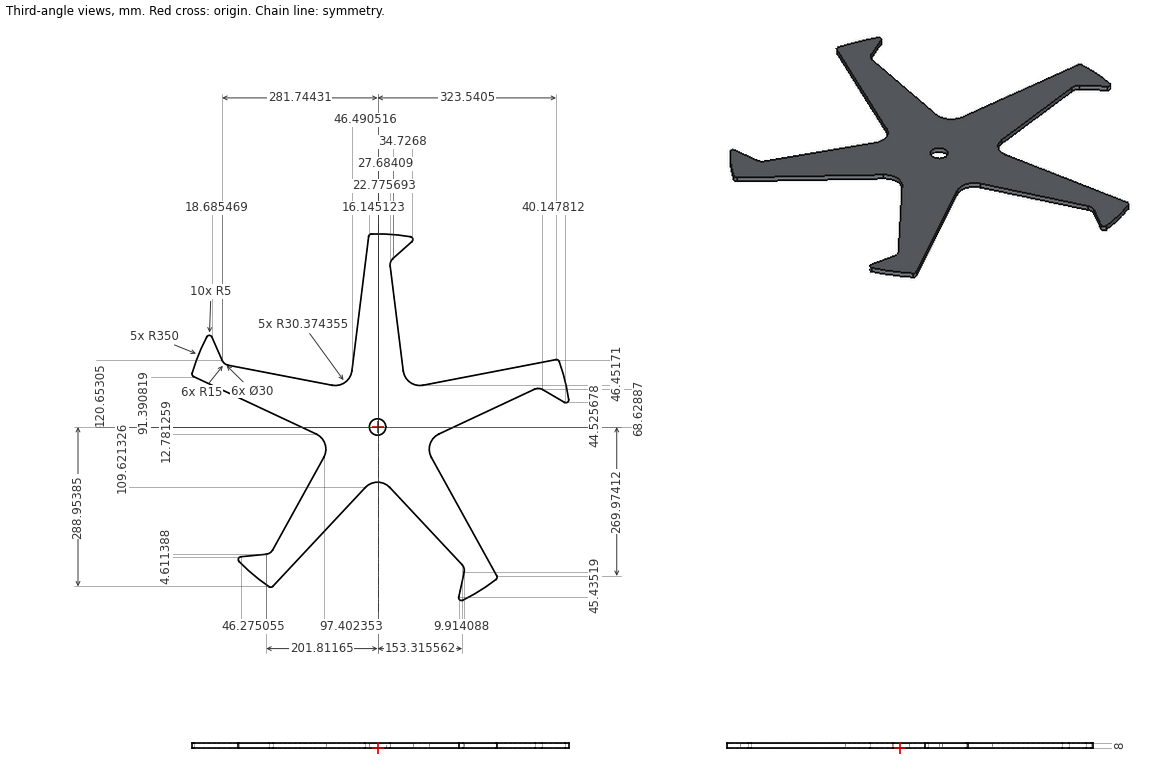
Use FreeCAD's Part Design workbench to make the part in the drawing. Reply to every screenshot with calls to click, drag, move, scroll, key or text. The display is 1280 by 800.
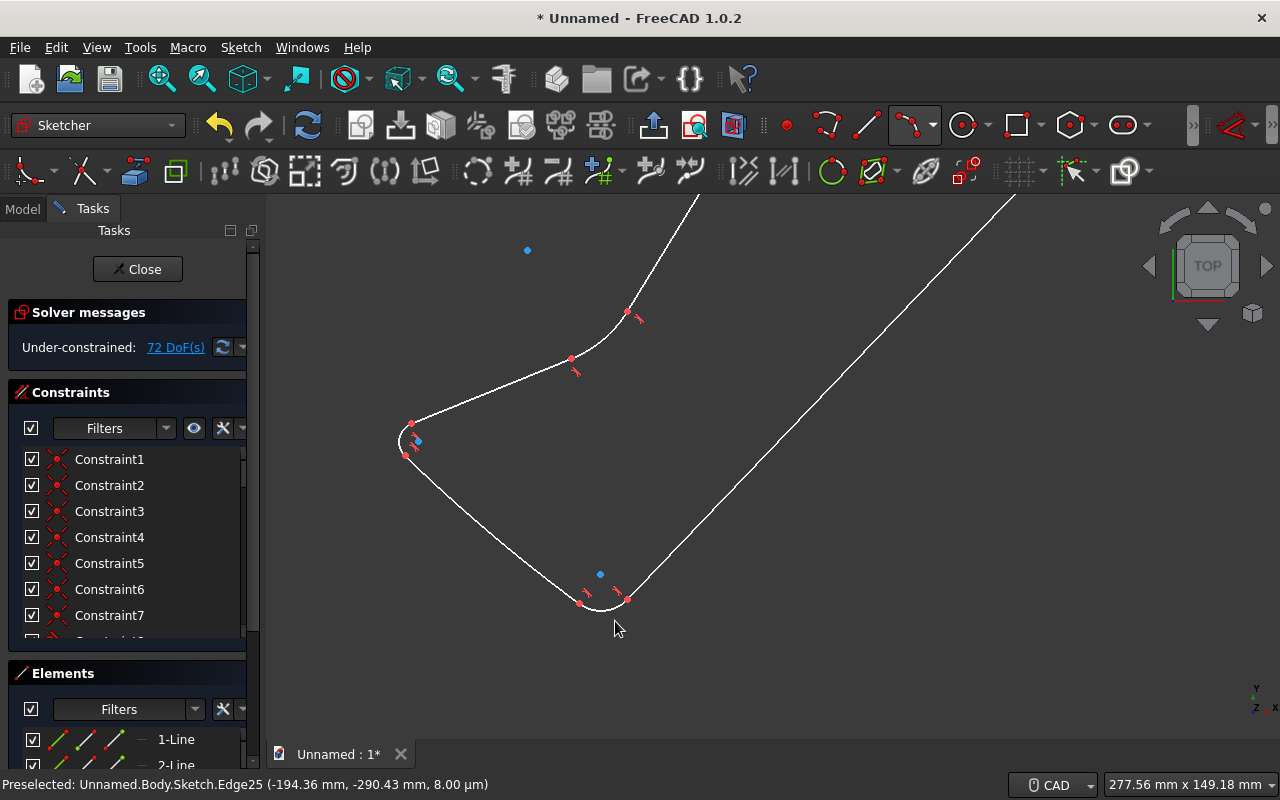
scroll(605, 618, down, 10)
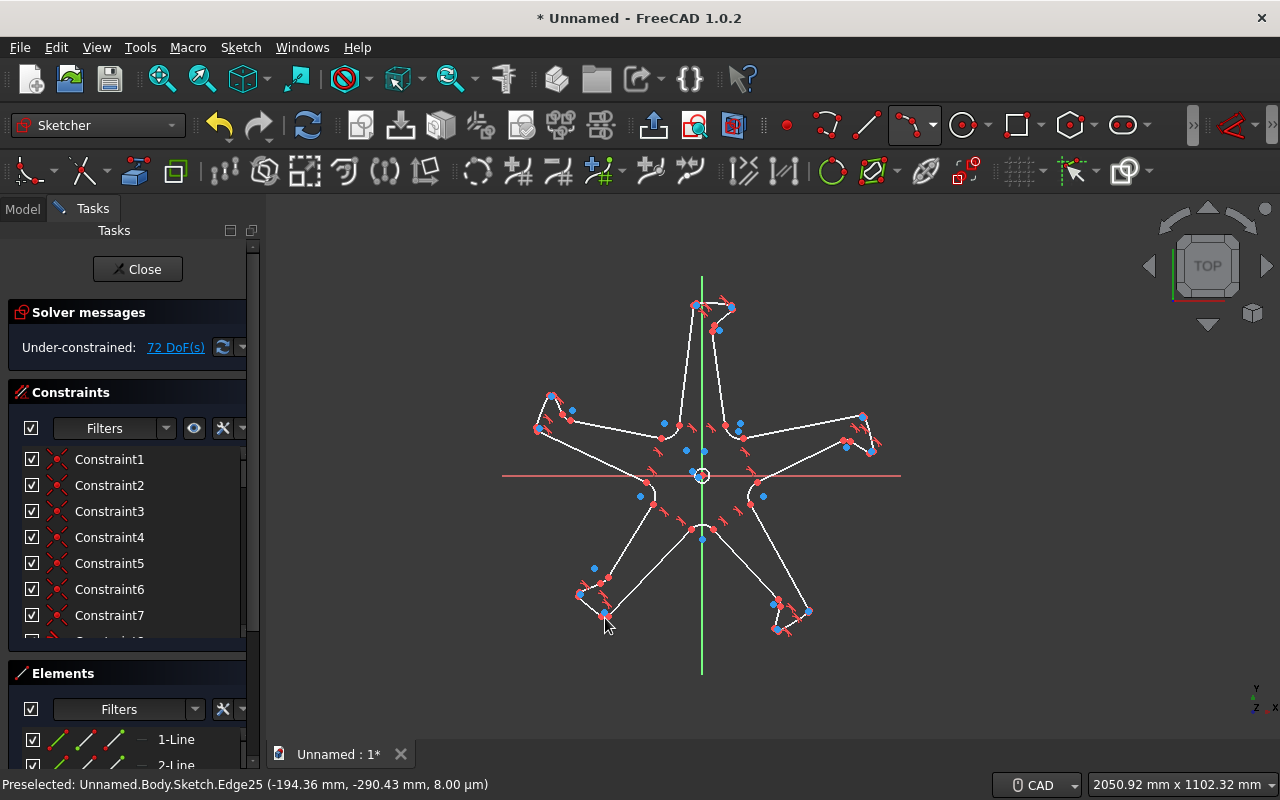
scroll(775, 630, up, 11)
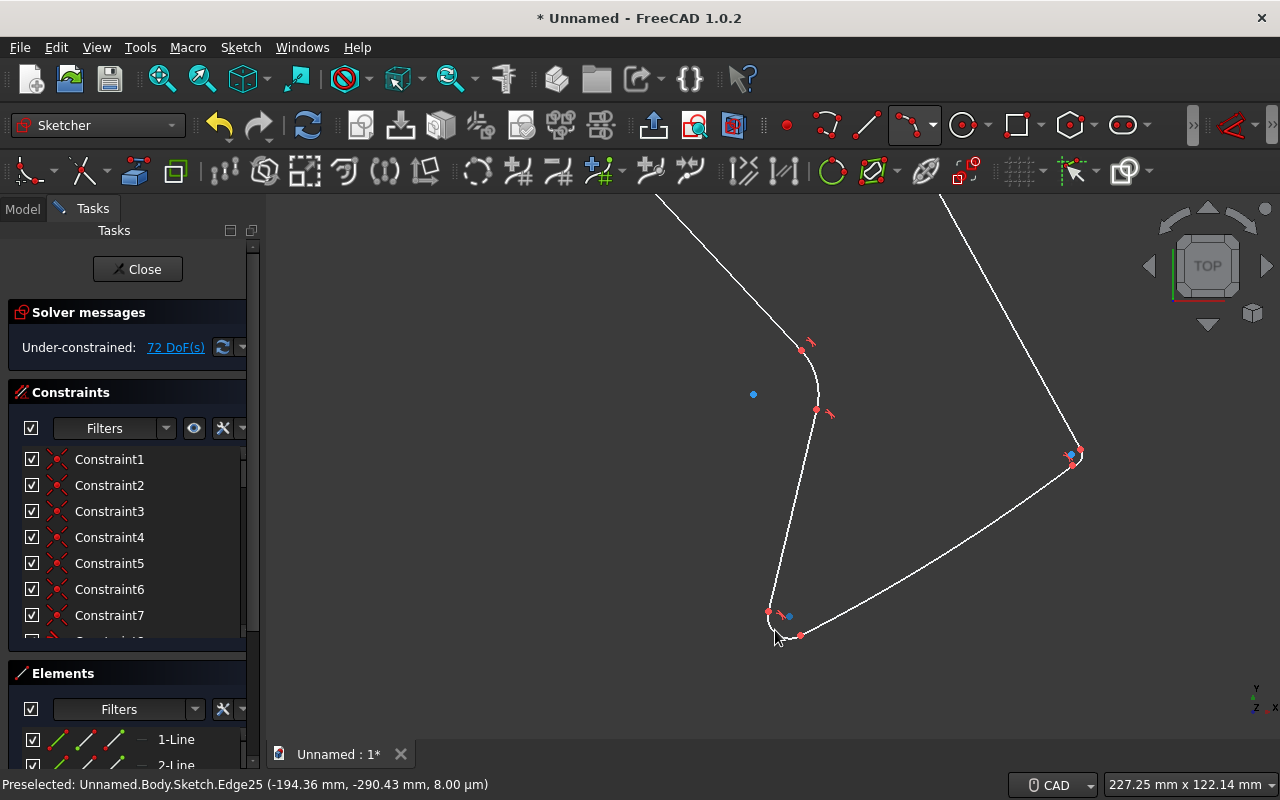
click(770, 627)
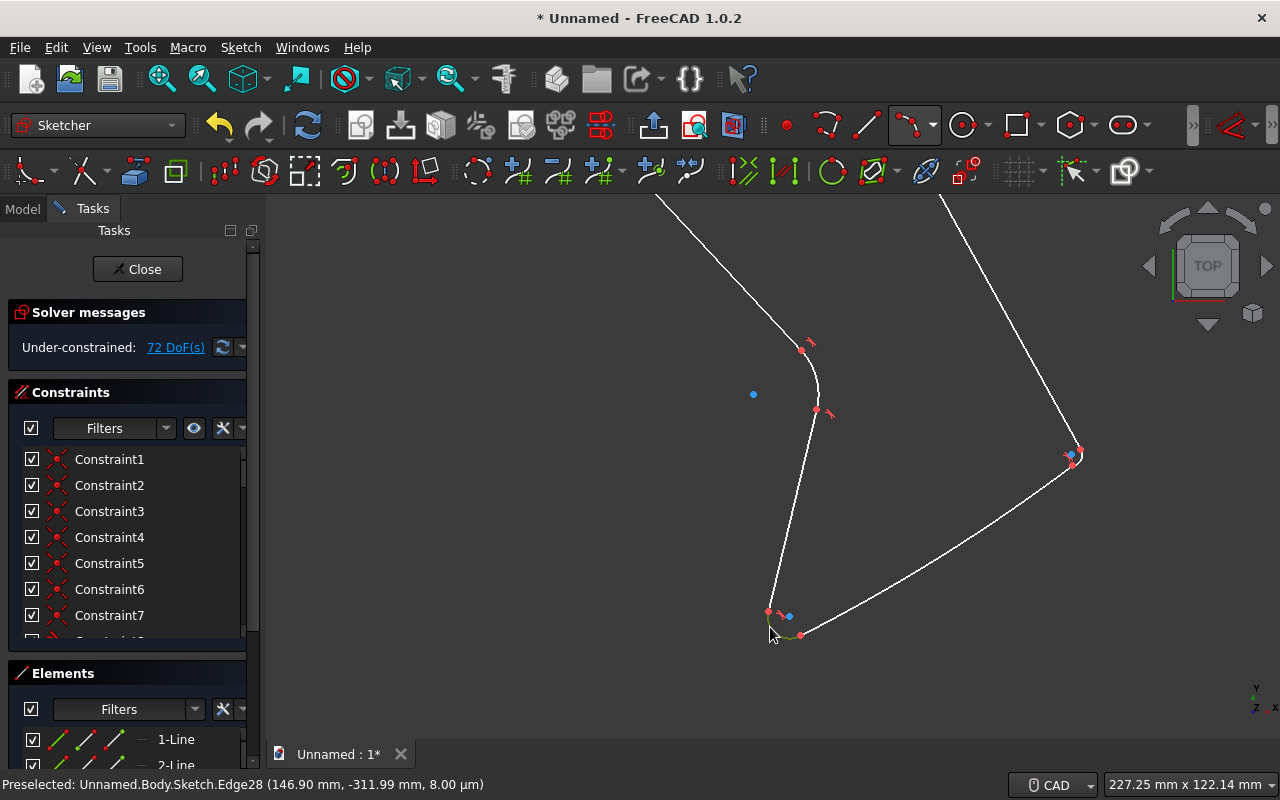
scroll(775, 630, down, 11)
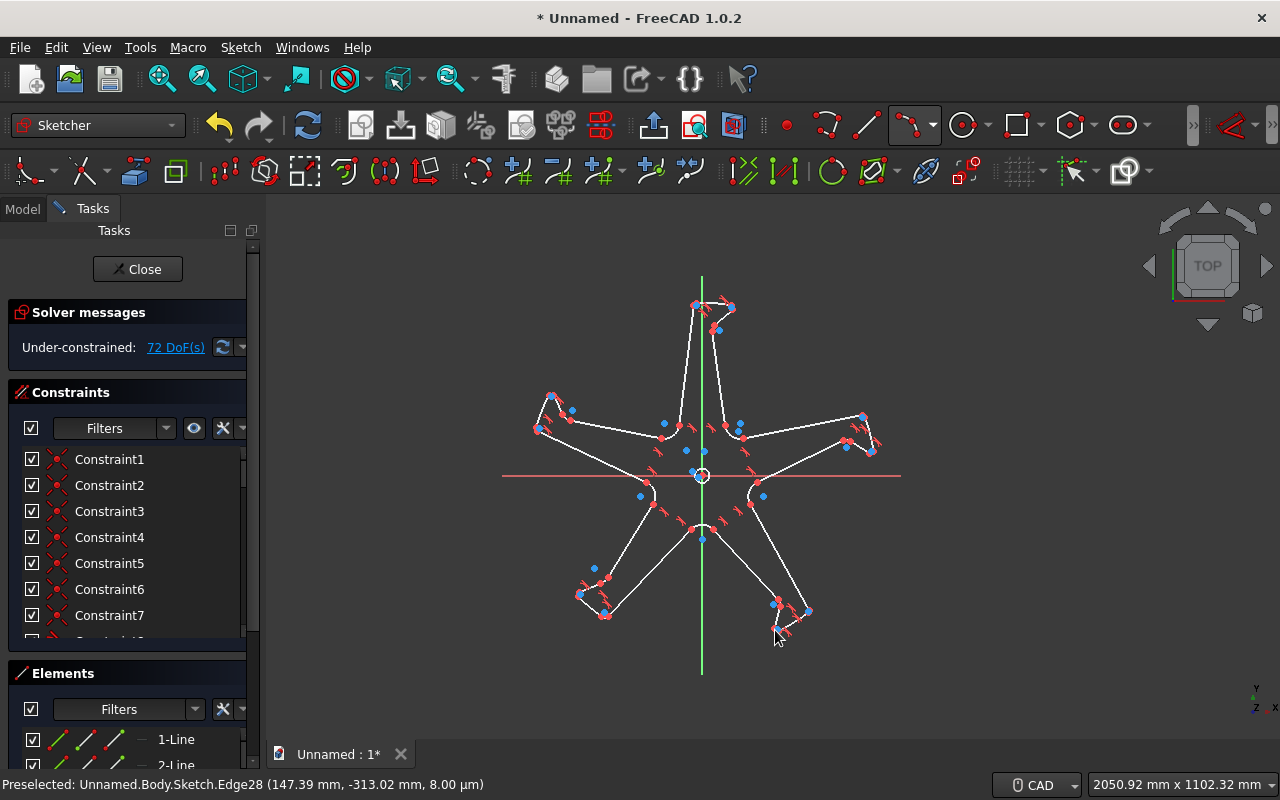
scroll(788, 626, up, 2)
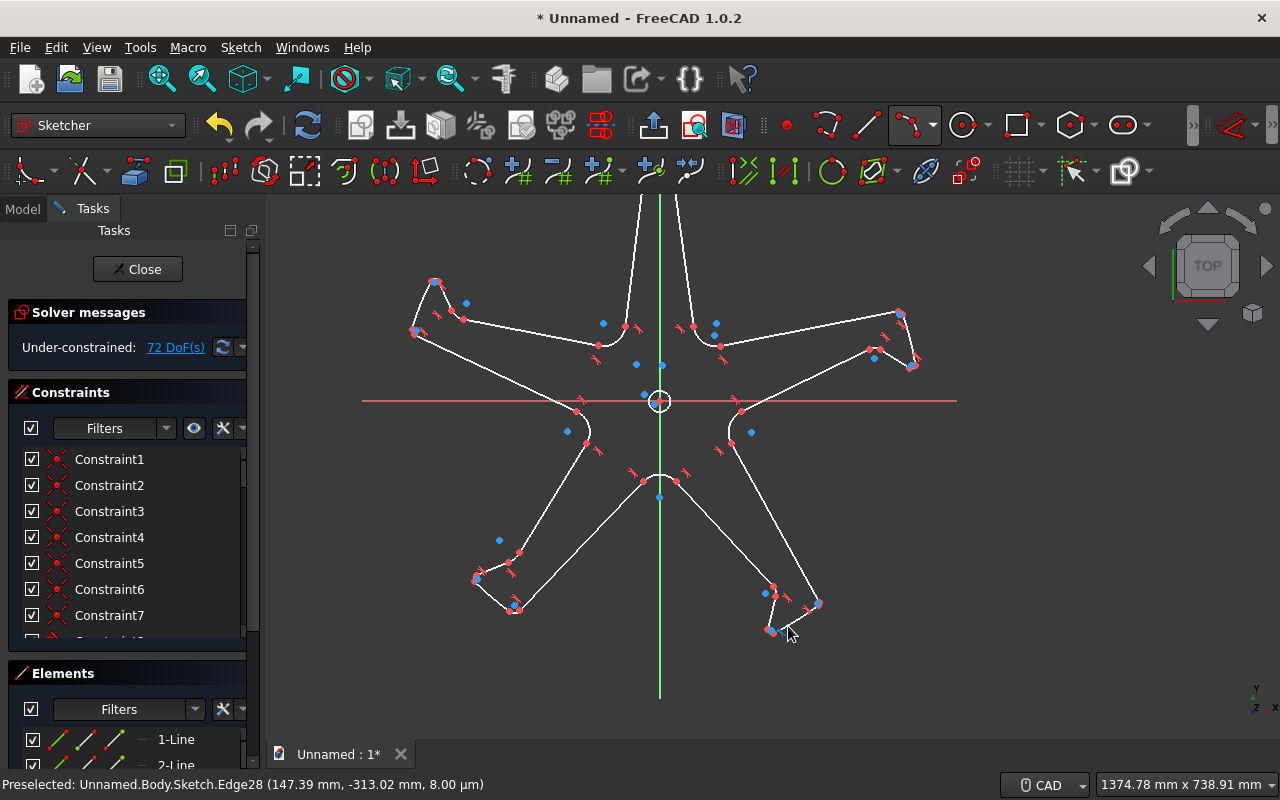
click(805, 615)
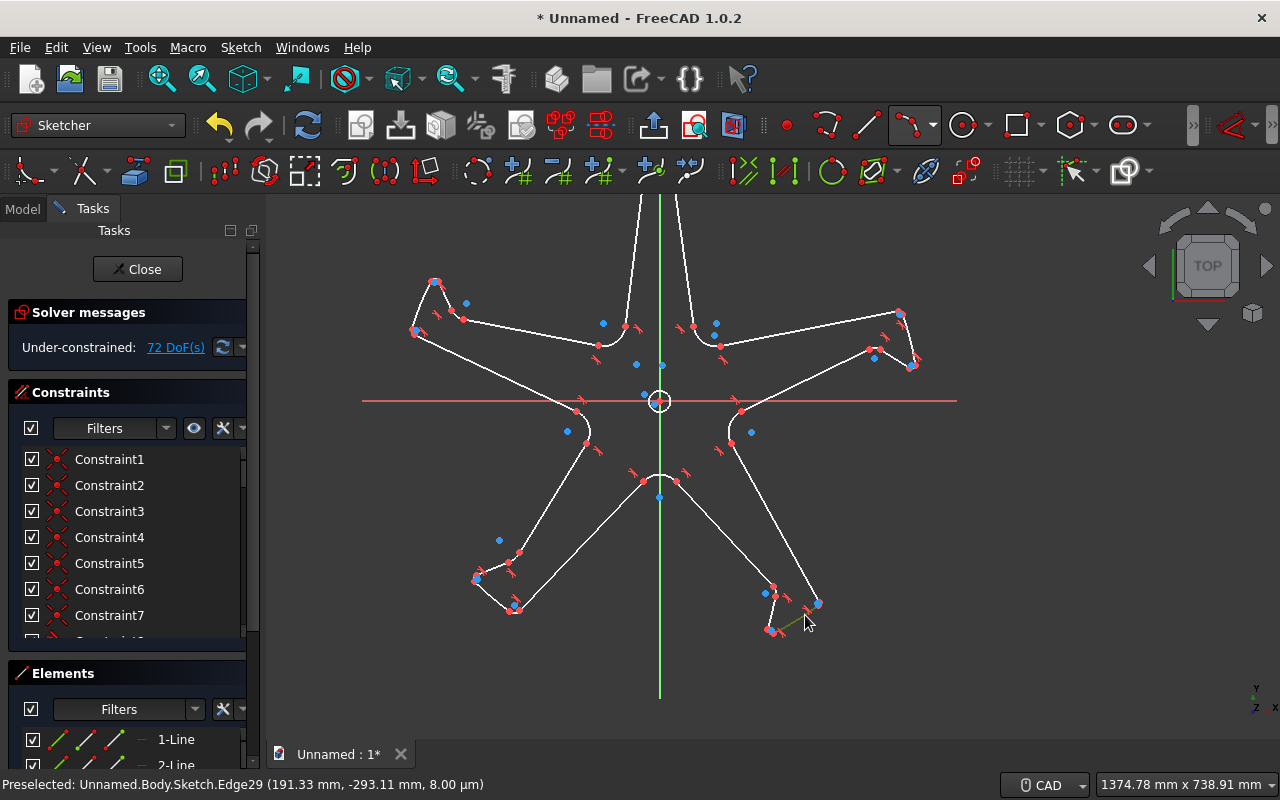
key(t)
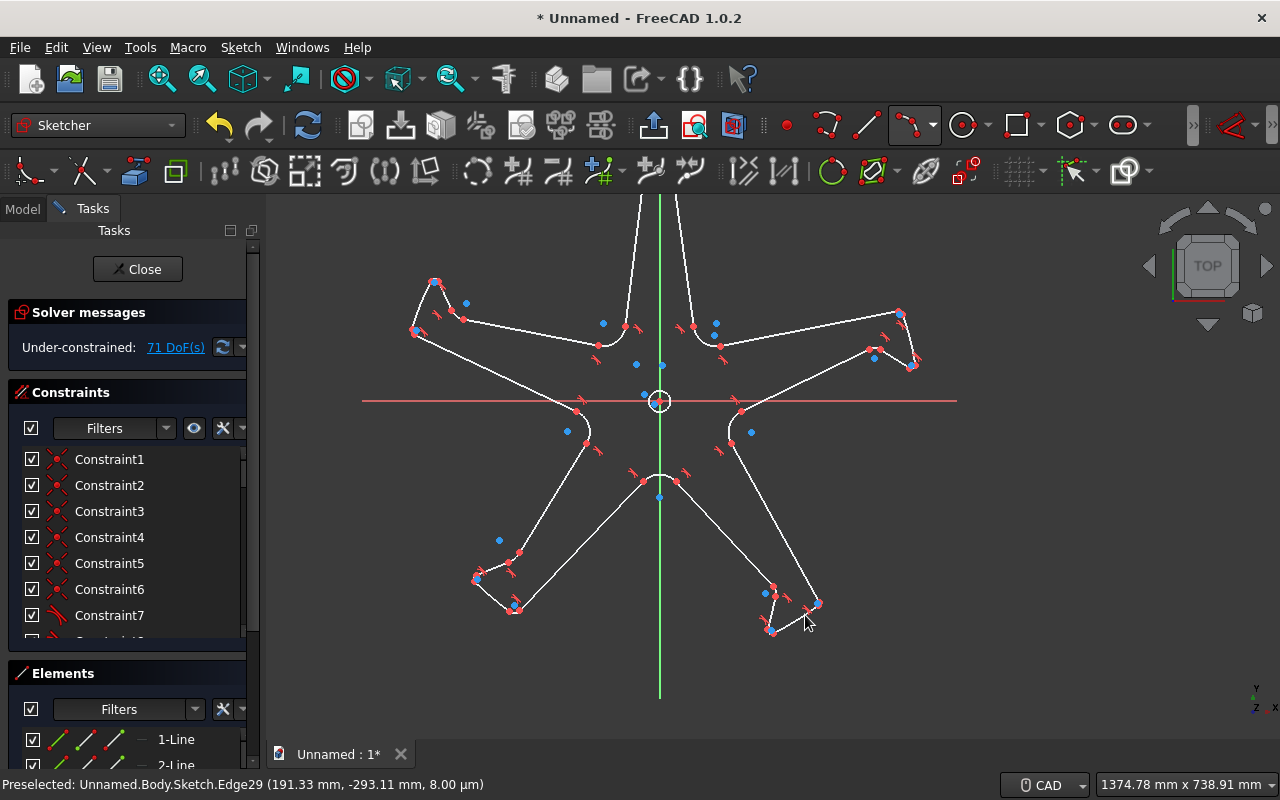
click(787, 626)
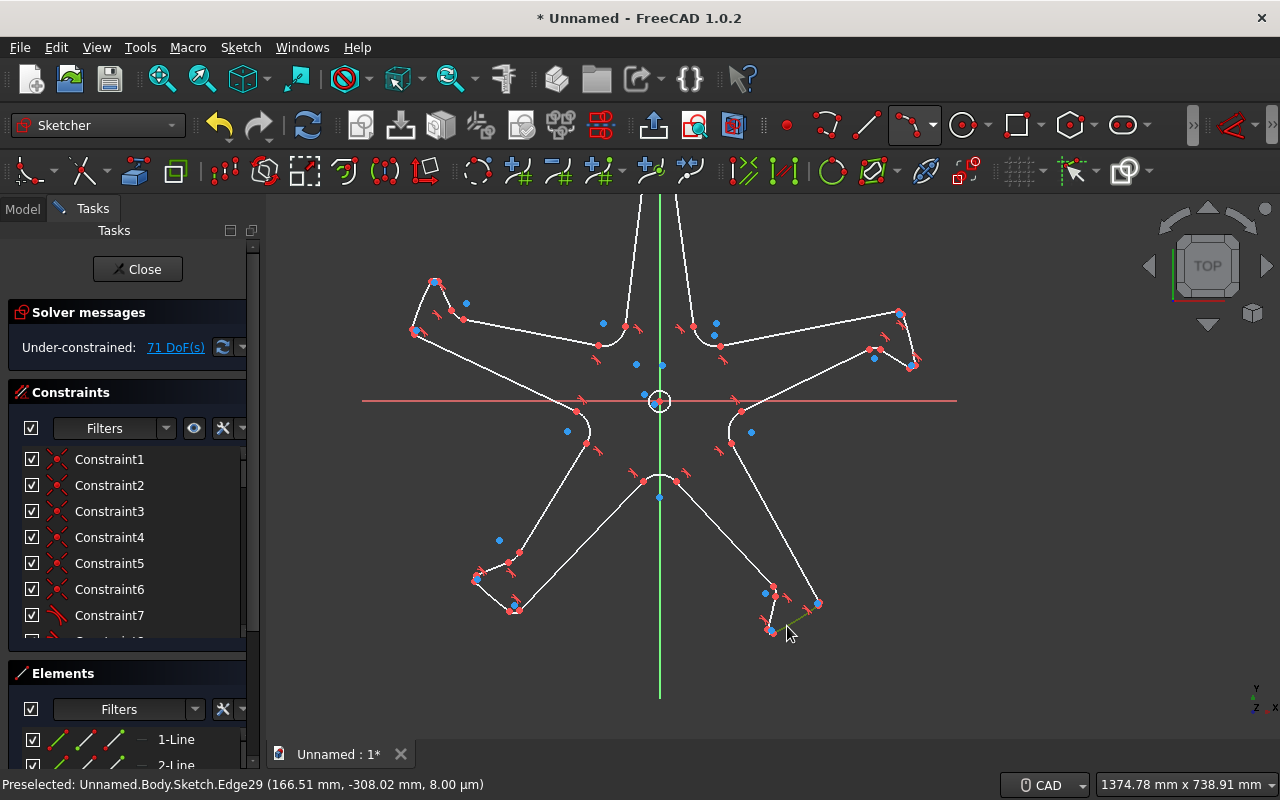
scroll(820, 605, up, 11)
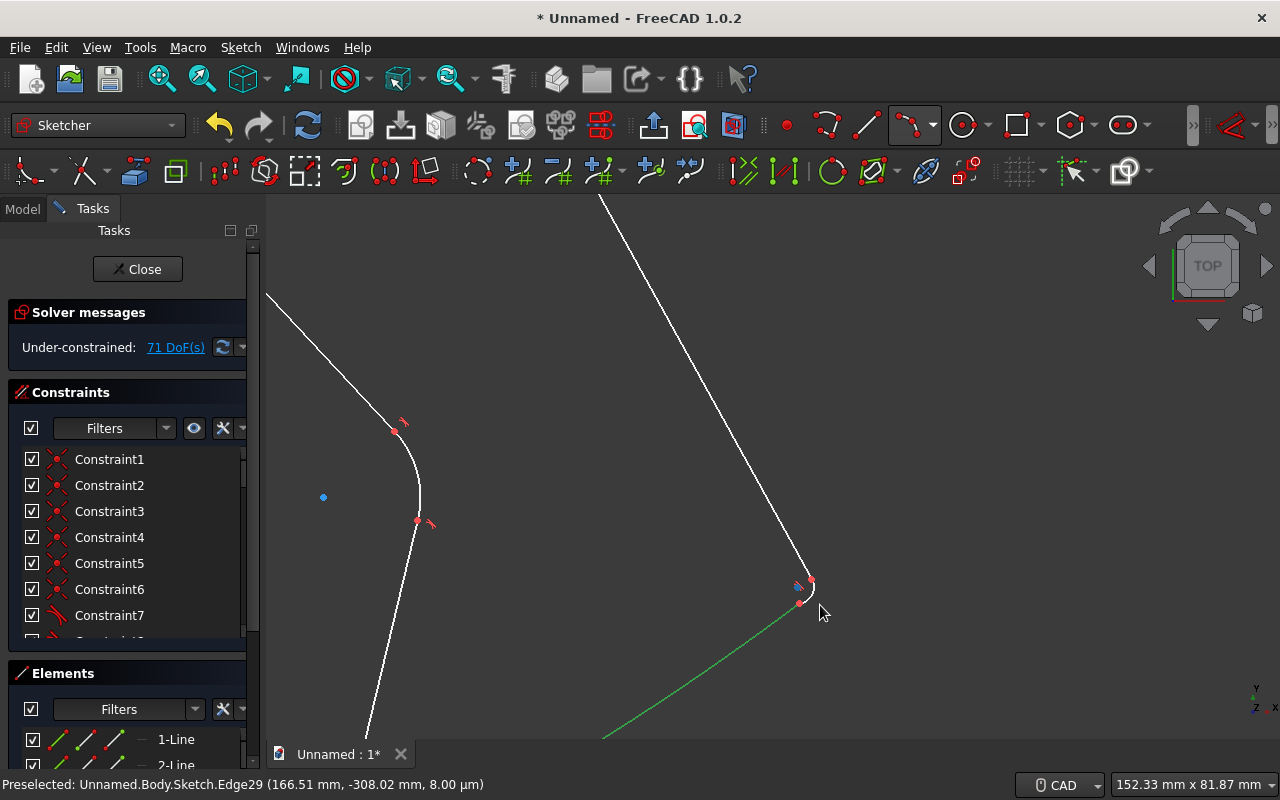
click(812, 595)